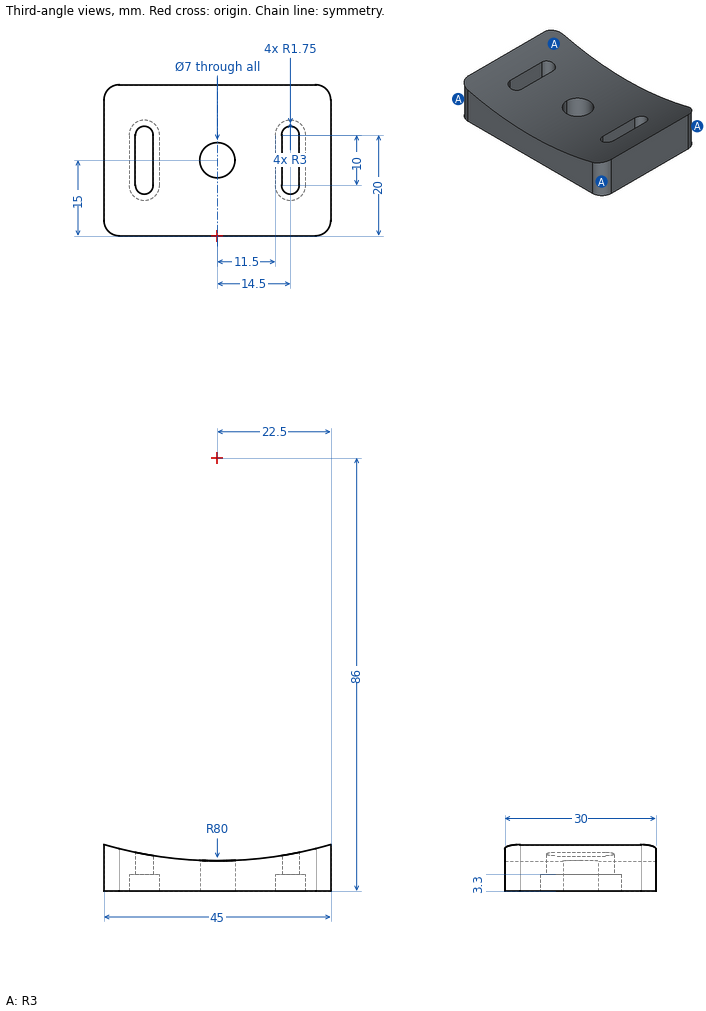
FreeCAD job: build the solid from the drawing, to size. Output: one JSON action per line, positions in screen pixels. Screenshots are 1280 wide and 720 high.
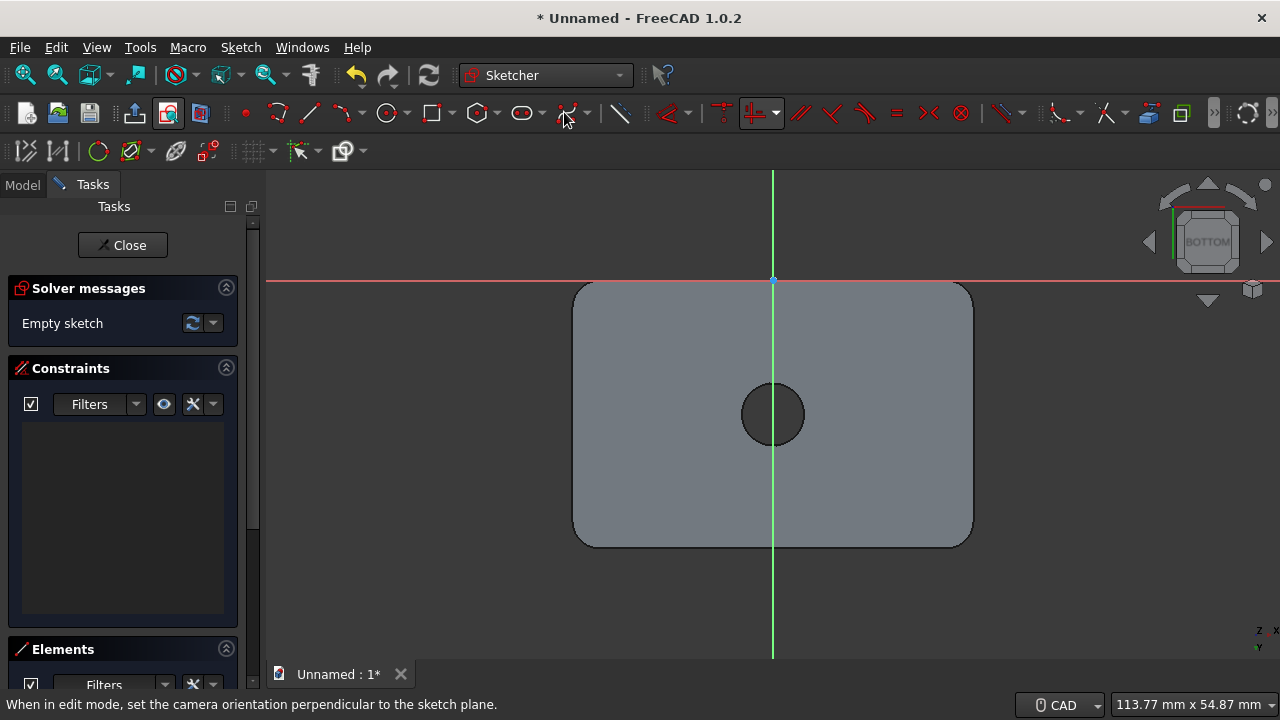
{"action": "scroll", "coordinate": [912, 303], "scroll_direction": "up", "scroll_amount": 2}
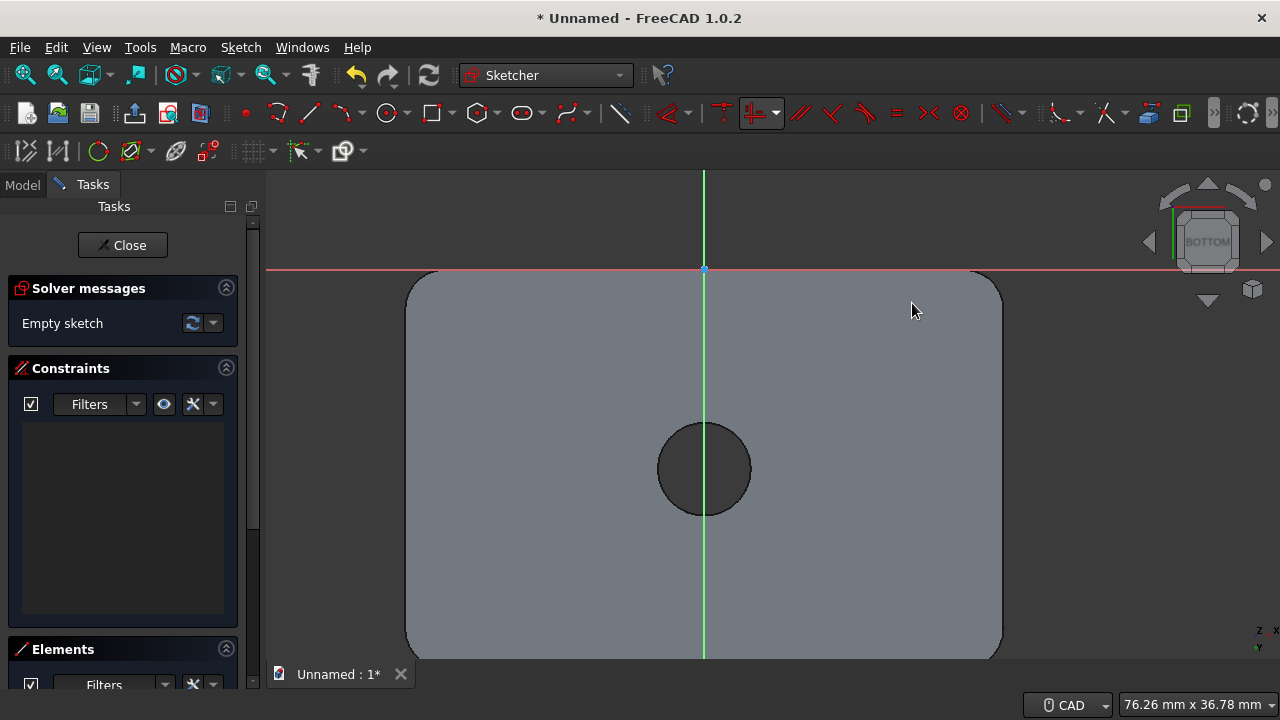
{"action": "key", "text": "g s"}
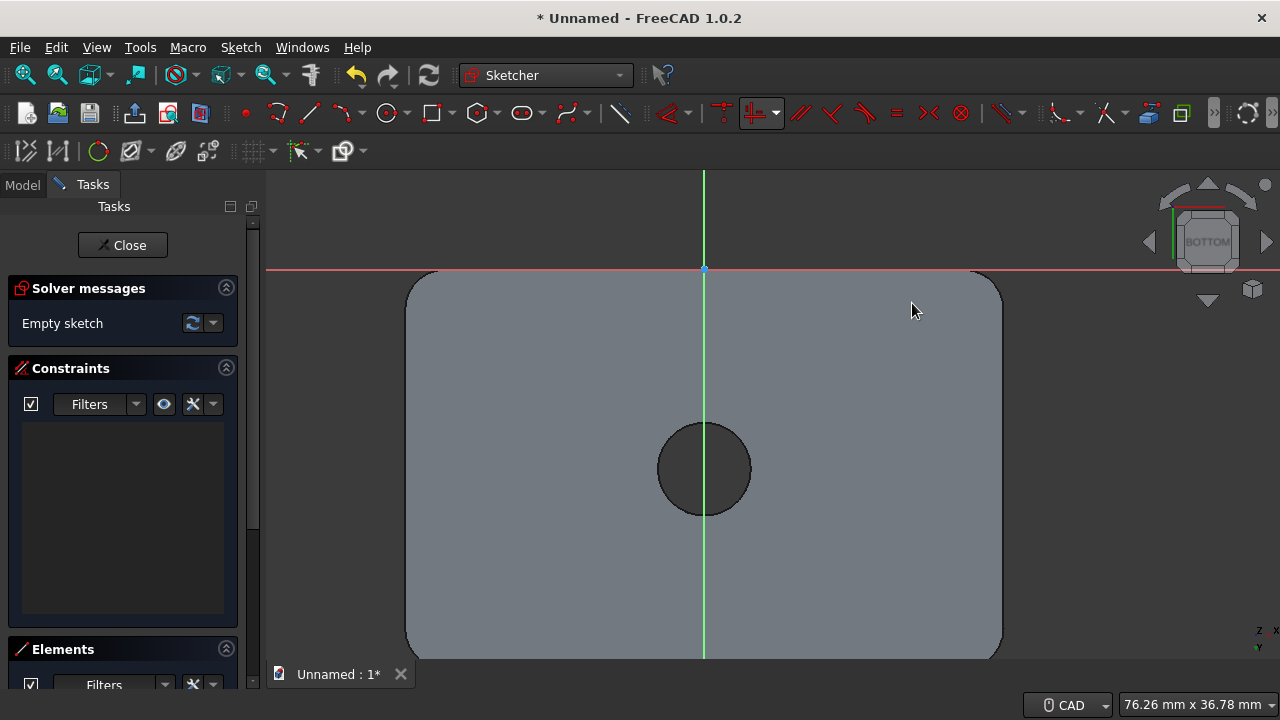
{"action": "left_click", "coordinate": [897, 536]}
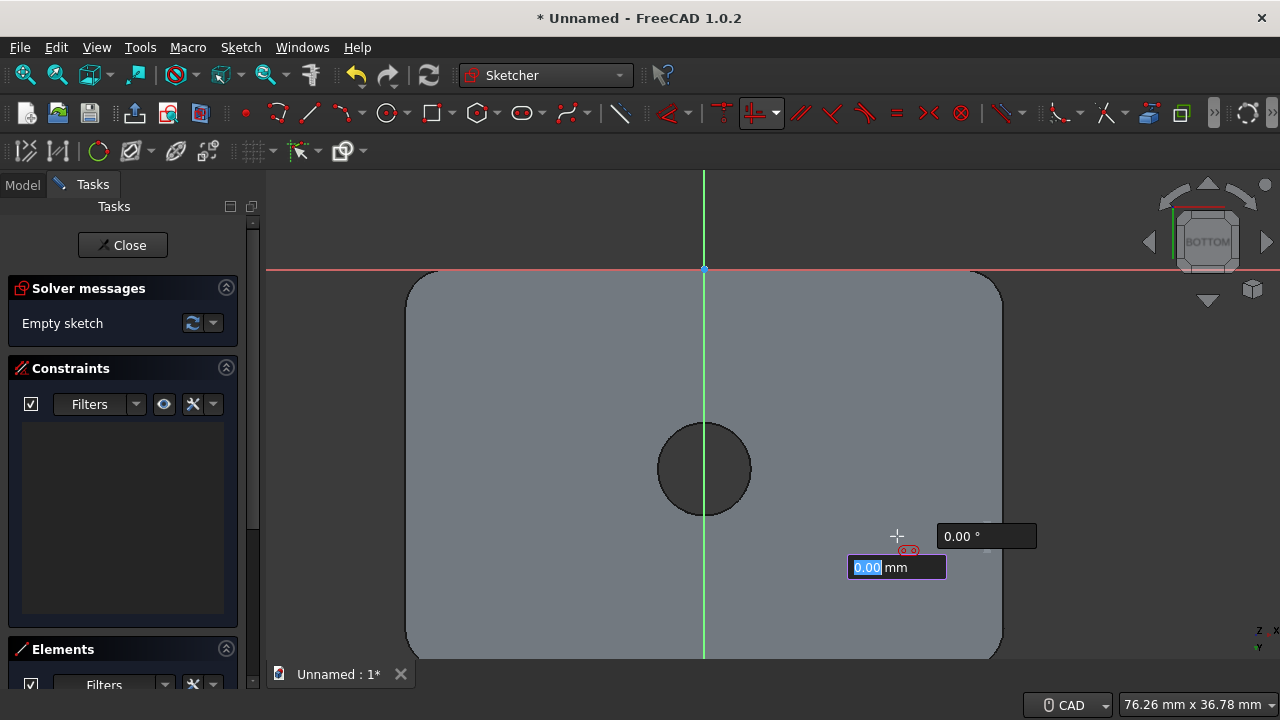
{"action": "left_click", "coordinate": [897, 403]}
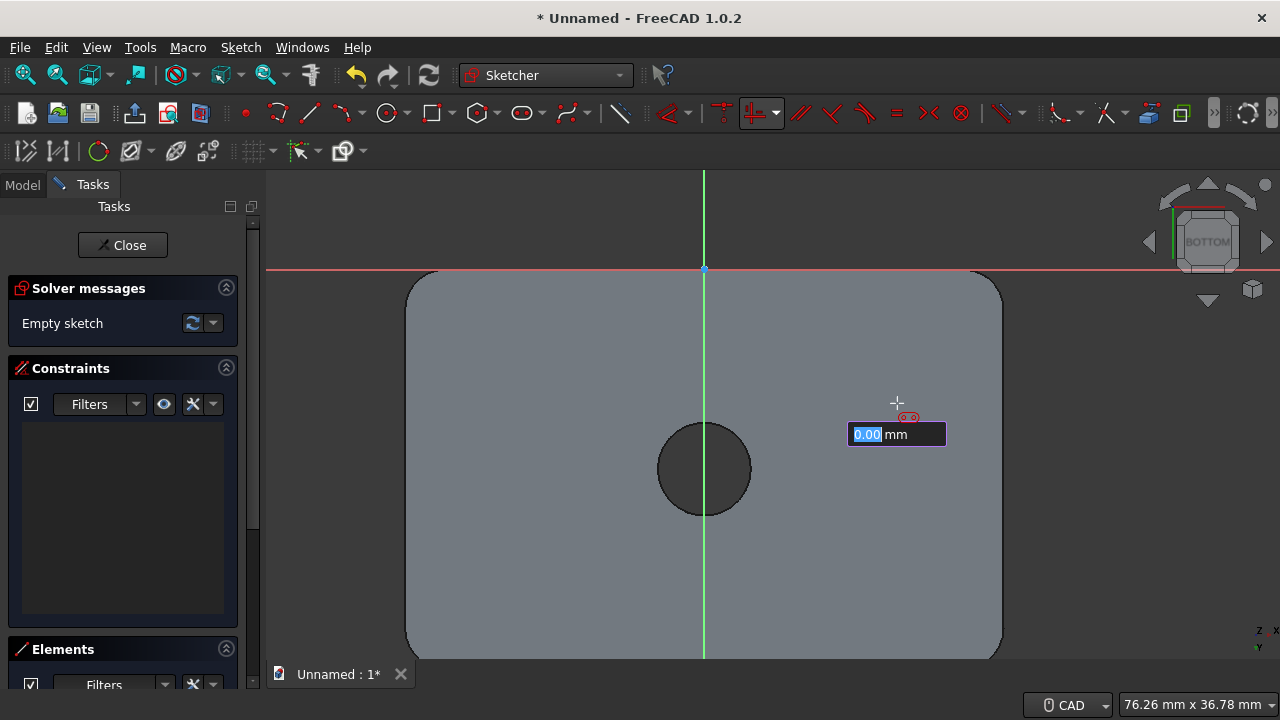
{"action": "left_click", "coordinate": [874, 469]}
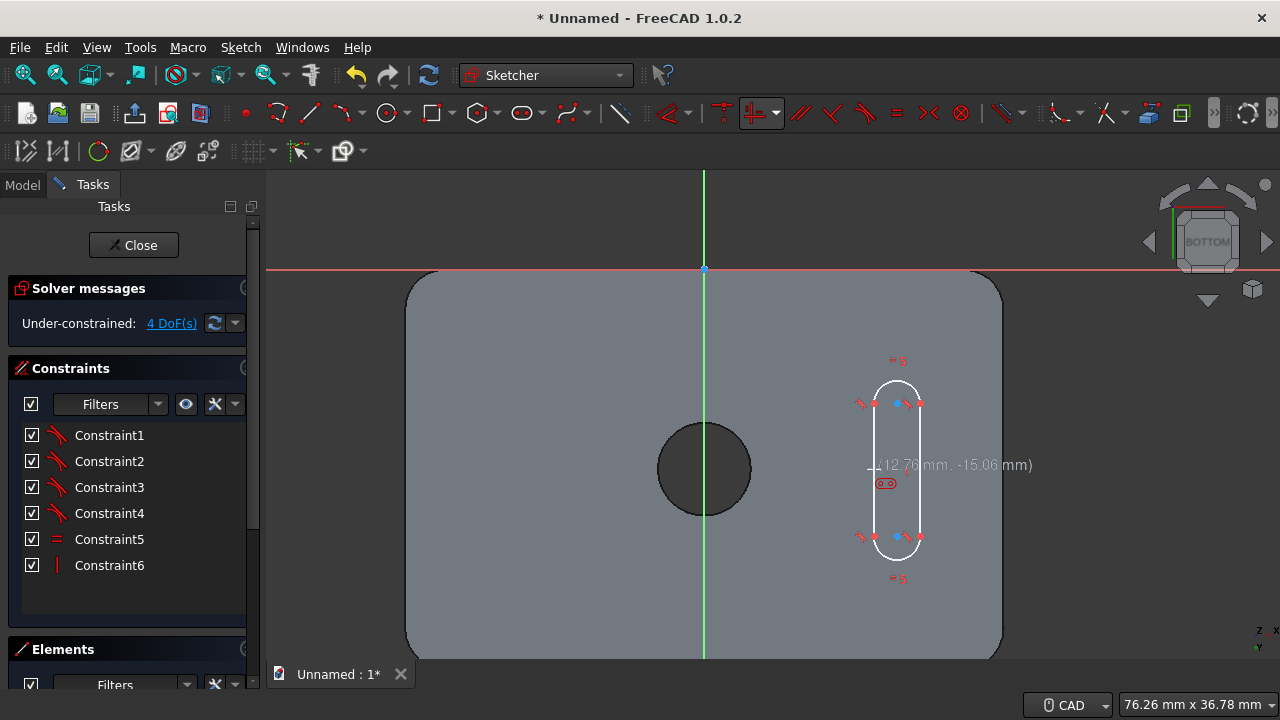
{"action": "left_click", "coordinate": [512, 536]}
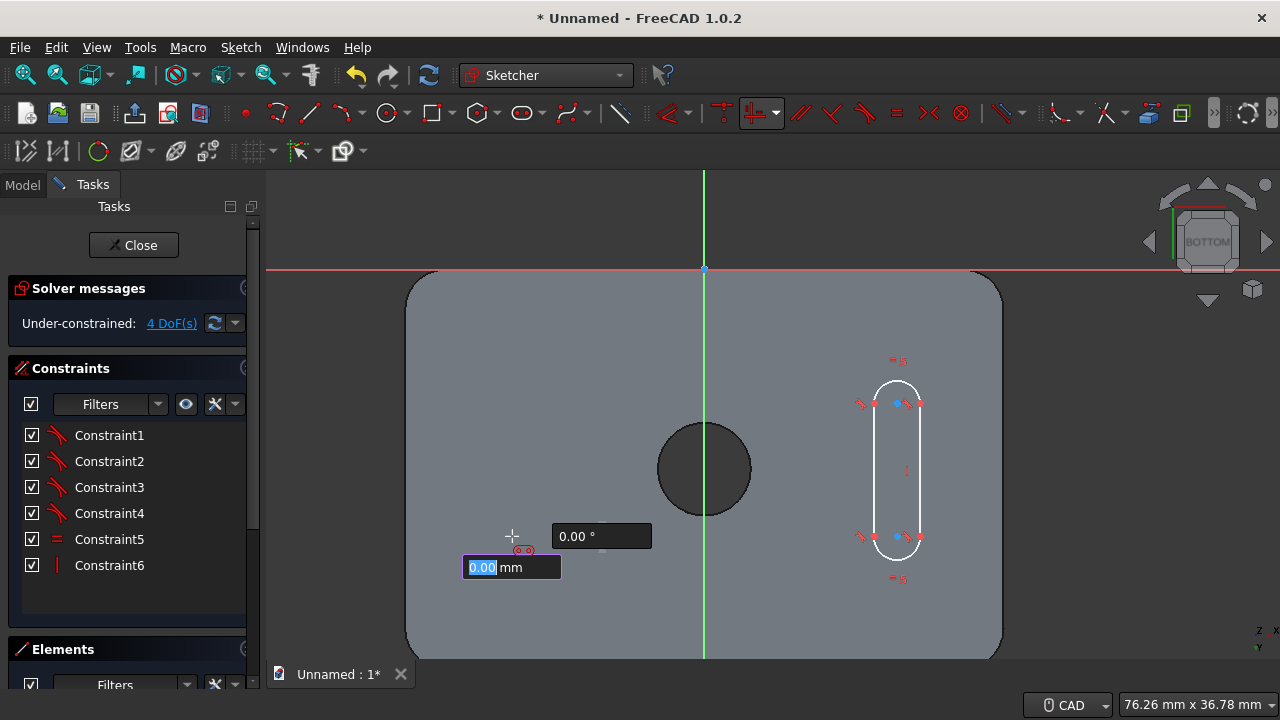
{"action": "left_click", "coordinate": [512, 403]}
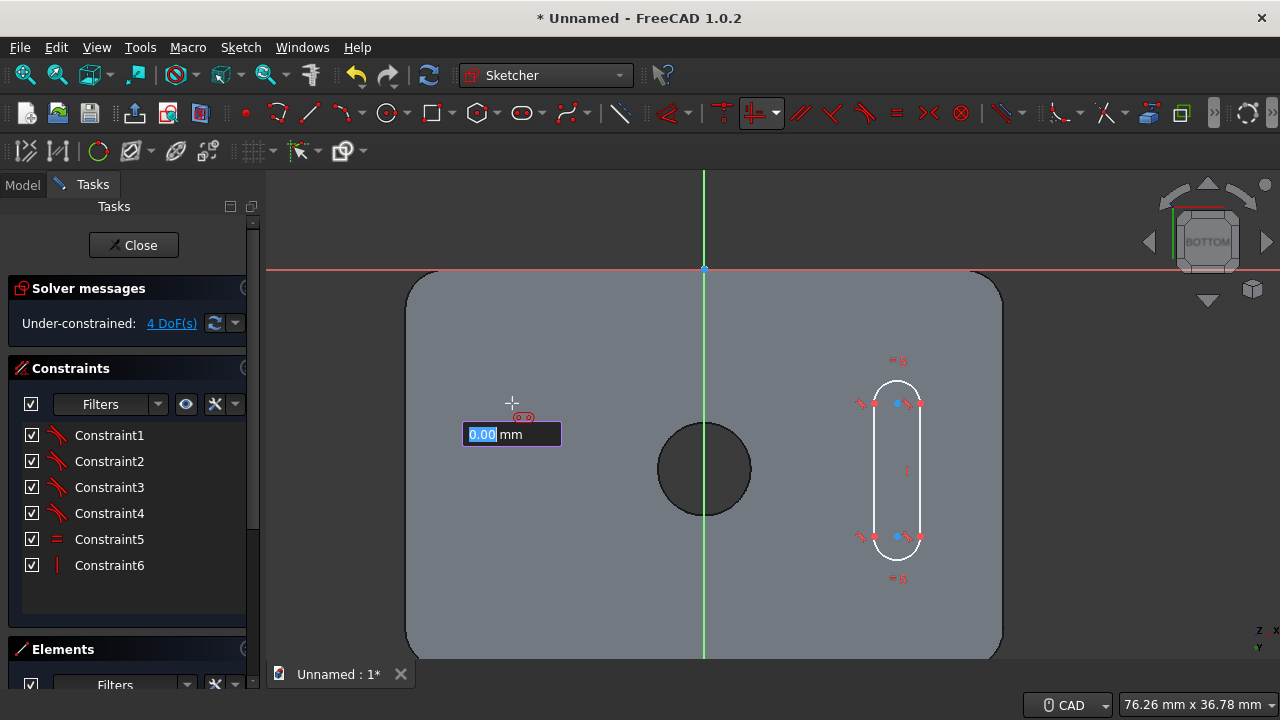
{"action": "left_click", "coordinate": [488, 469]}
{"action": "key", "text": "Escape"}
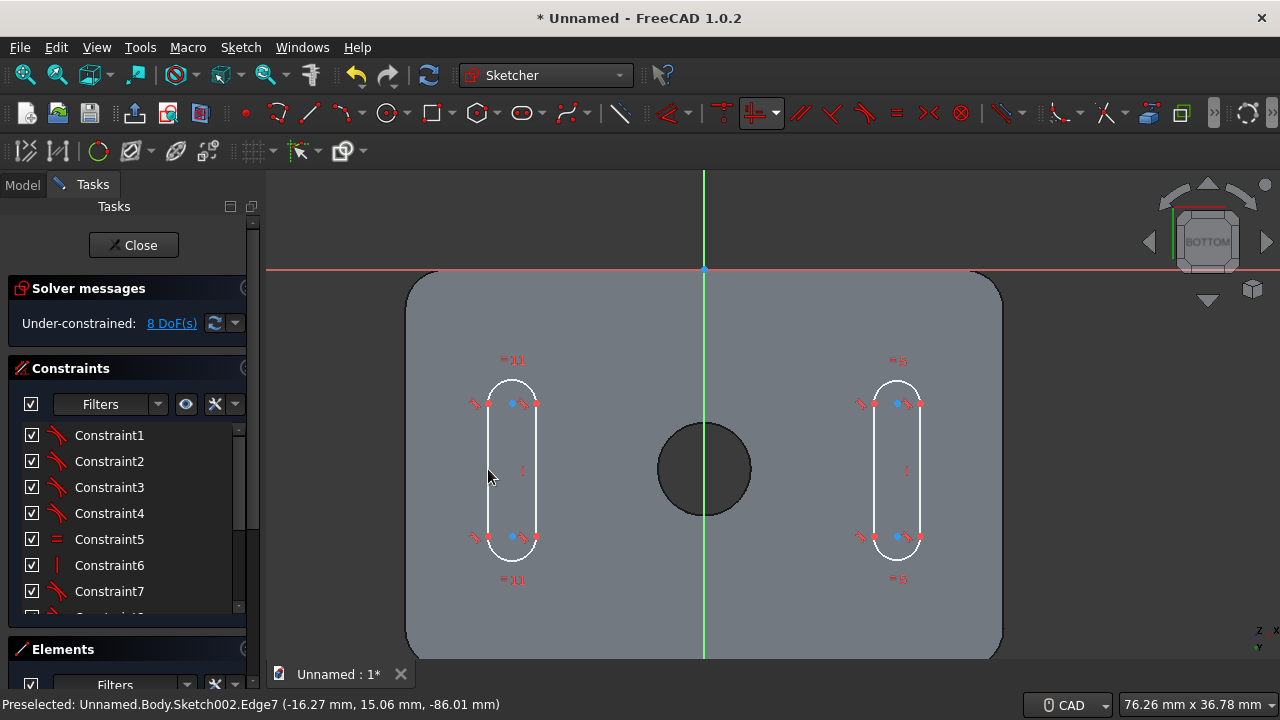
{"action": "left_click", "coordinate": [883, 556]}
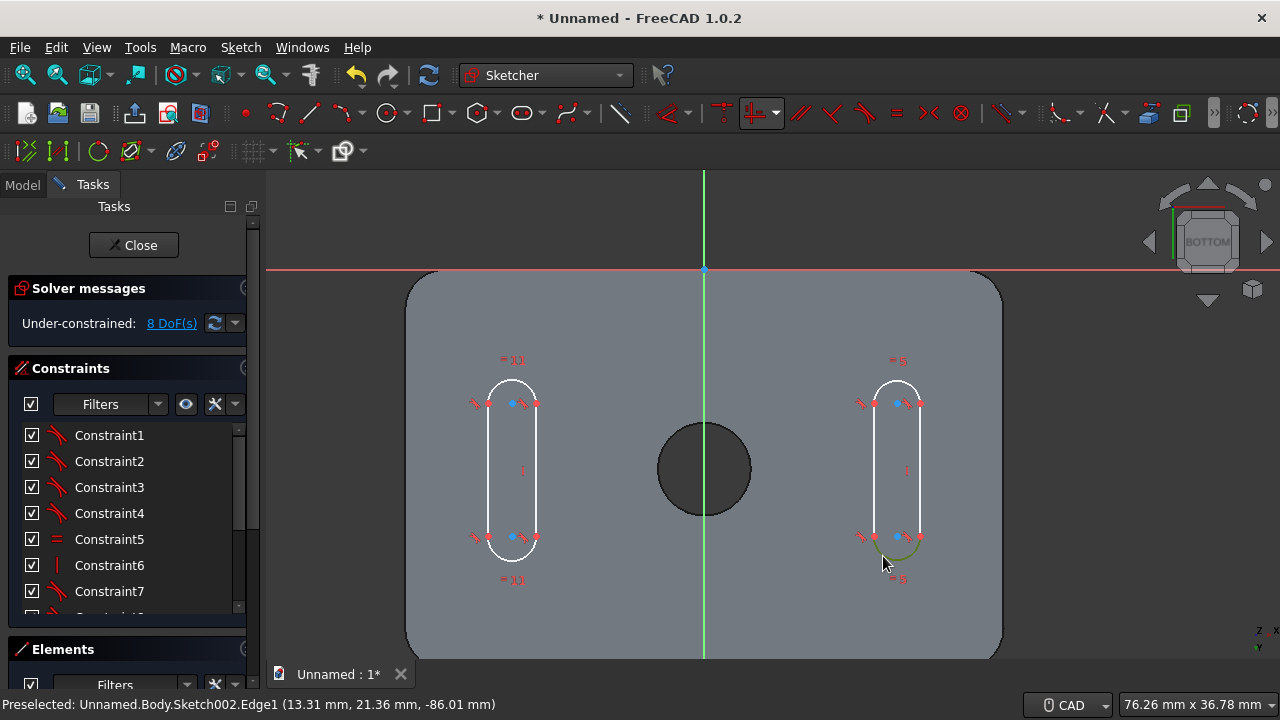
{"action": "left_click", "coordinate": [498, 556]}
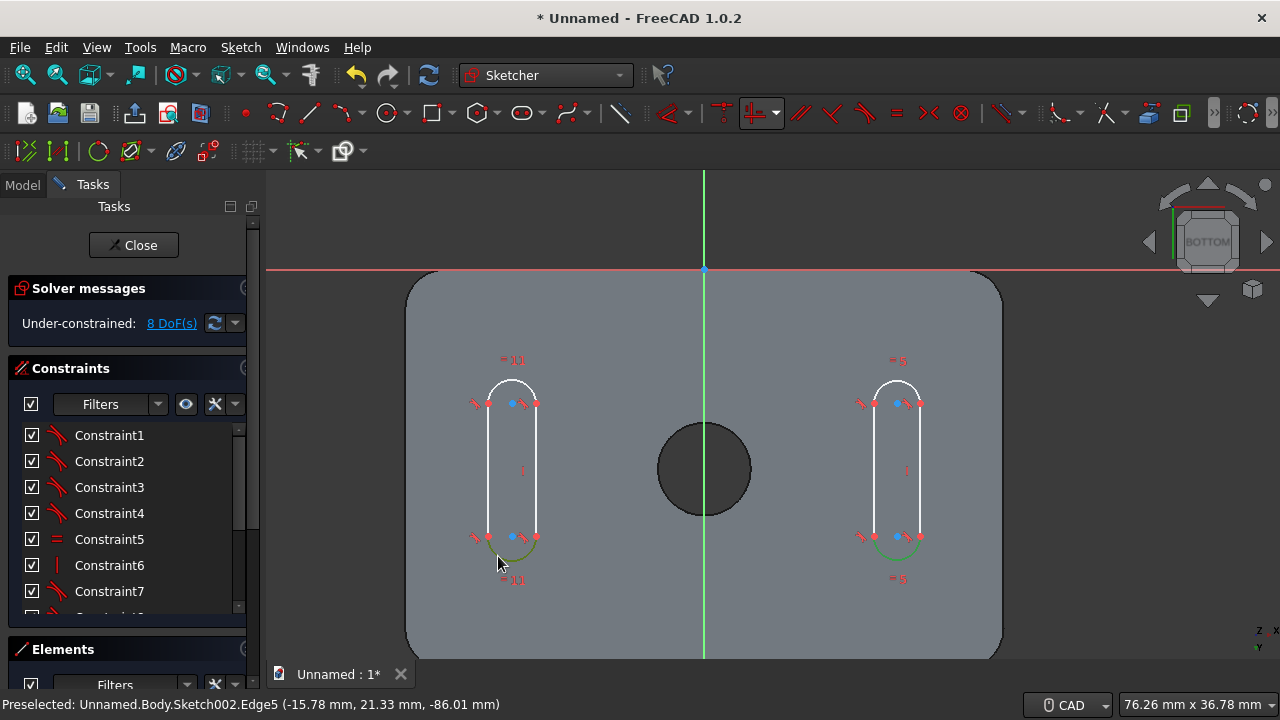
{"action": "left_click", "coordinate": [898, 114]}